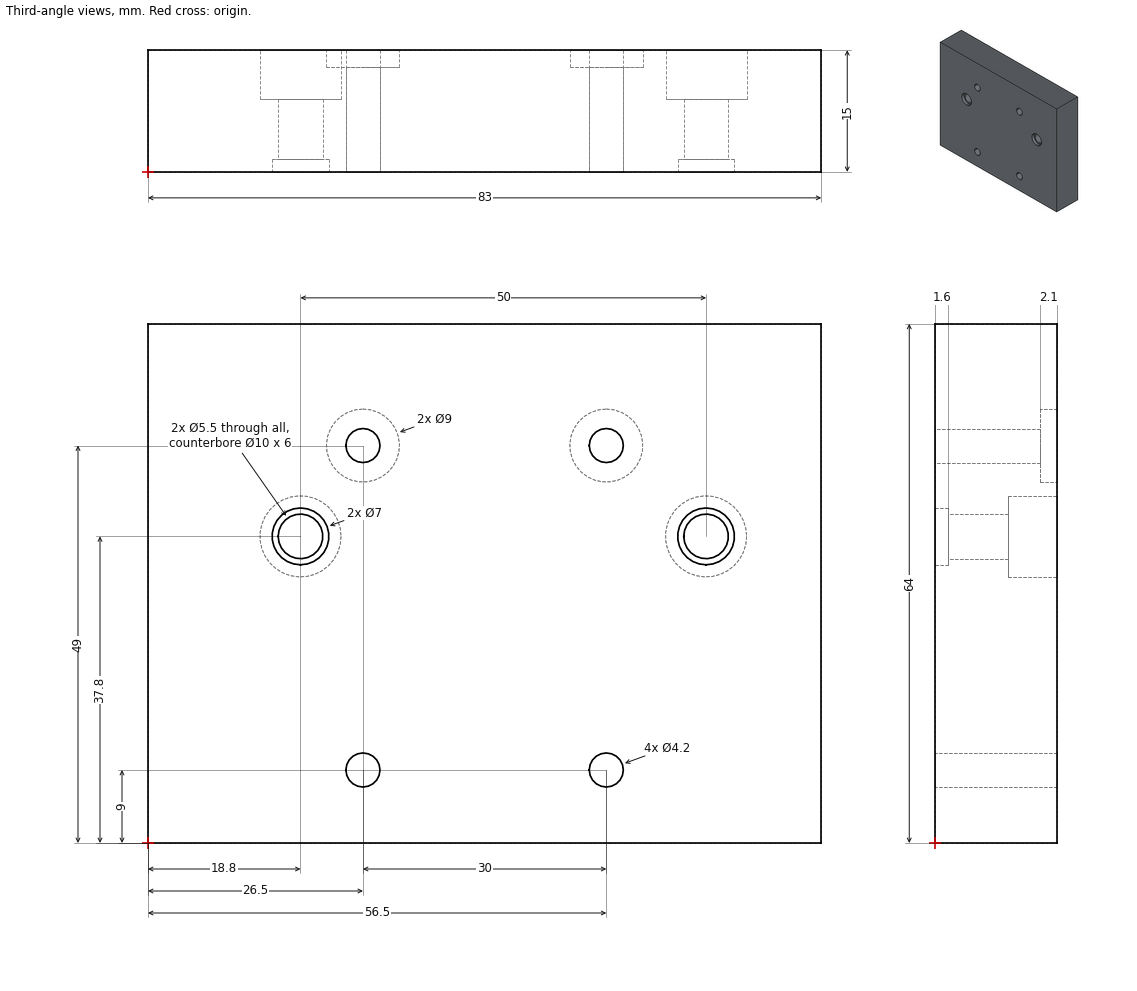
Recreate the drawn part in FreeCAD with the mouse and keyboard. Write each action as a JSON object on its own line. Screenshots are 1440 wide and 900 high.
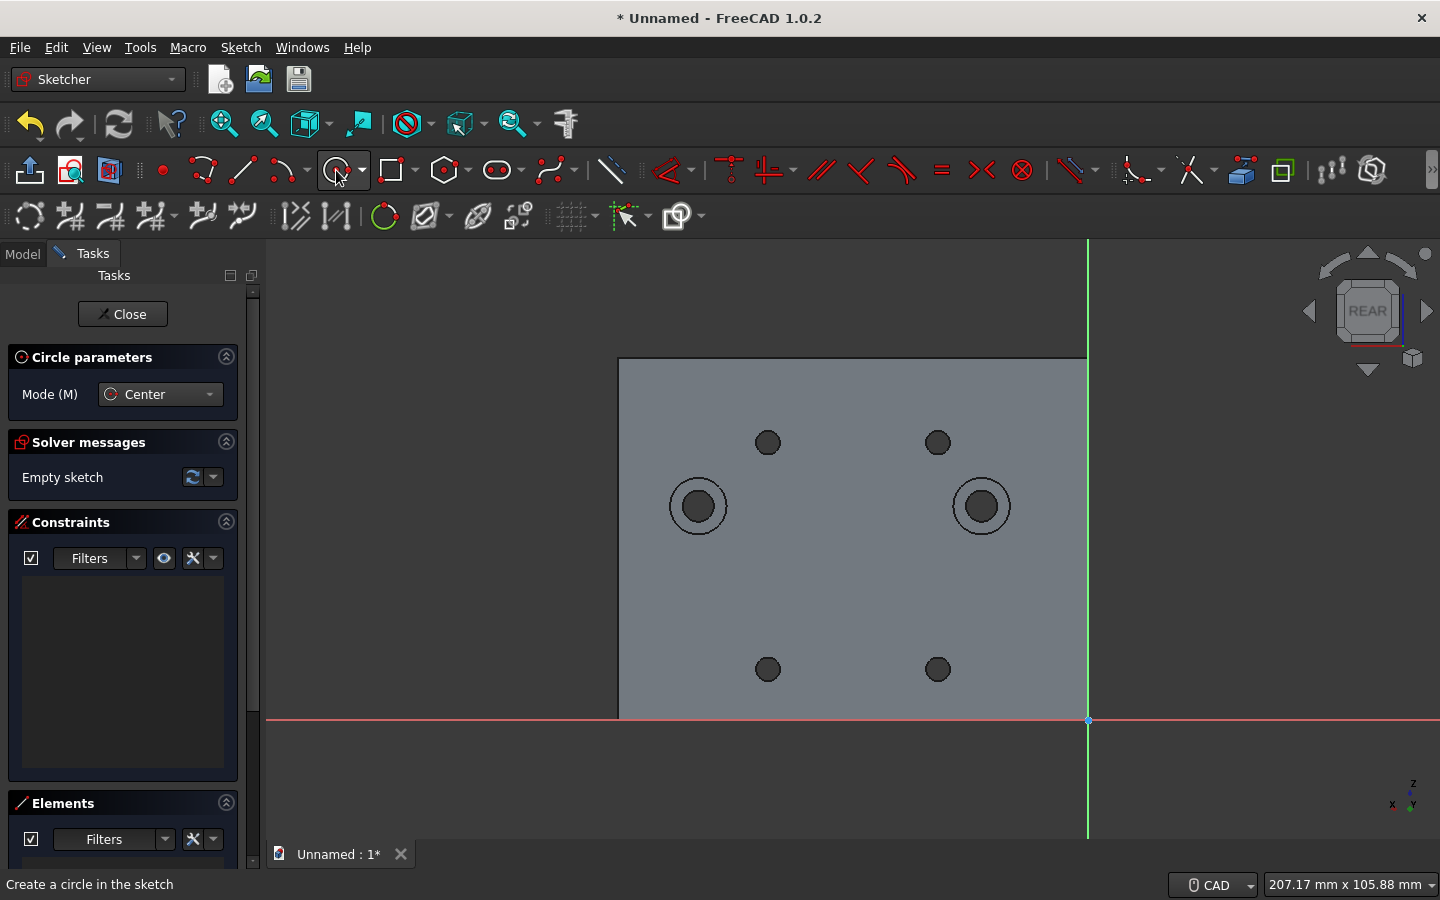
{"action": "left_click", "coordinate": [938, 443]}
{"action": "left_click", "coordinate": [956, 425]}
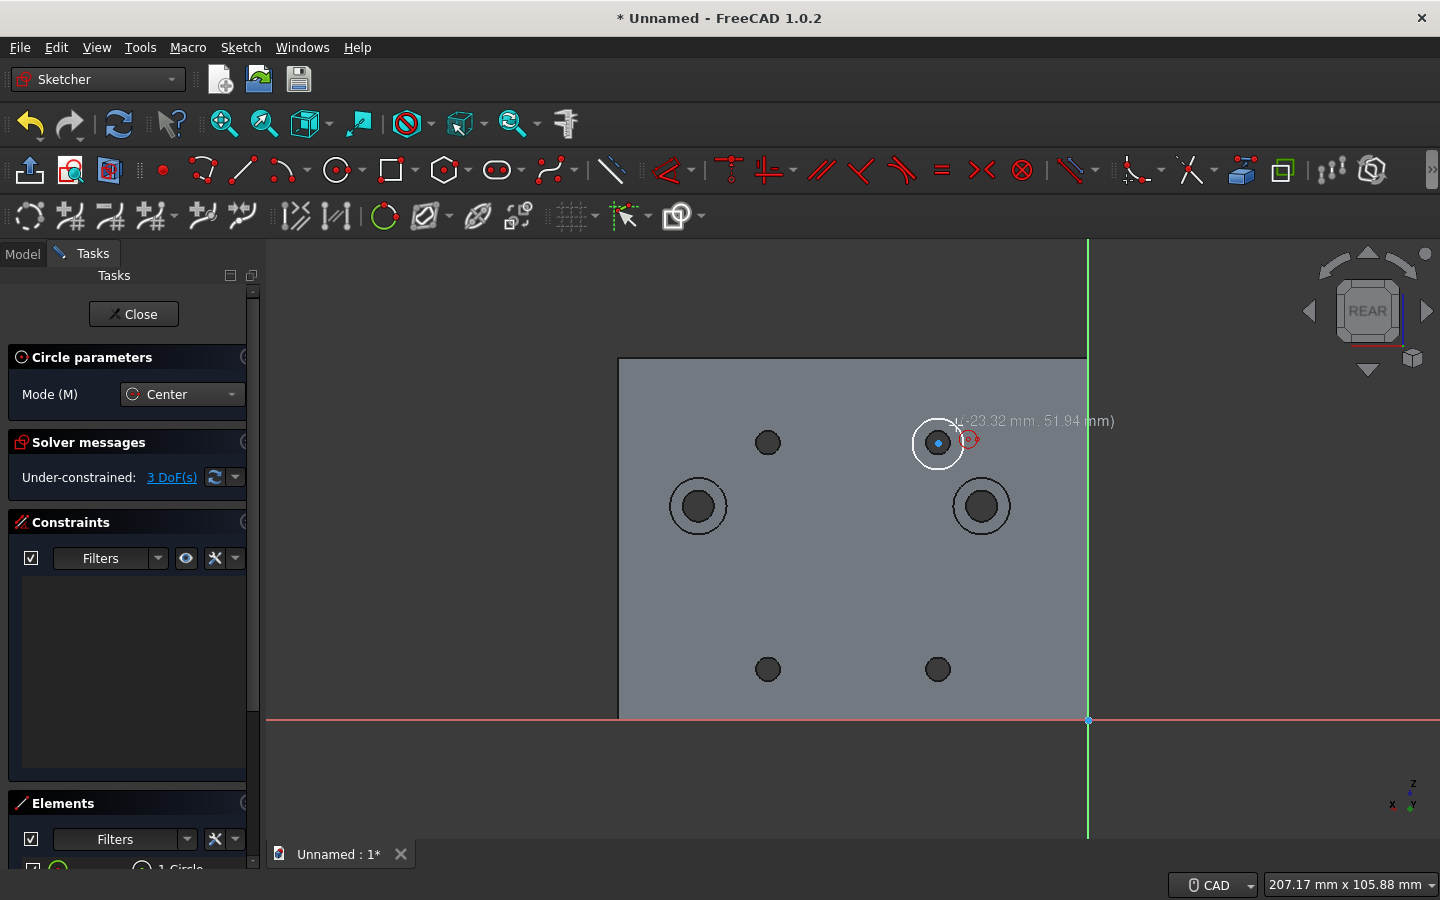
{"action": "left_click", "coordinate": [768, 443]}
{"action": "left_click", "coordinate": [786, 425]}
{"action": "key", "text": "Escape"}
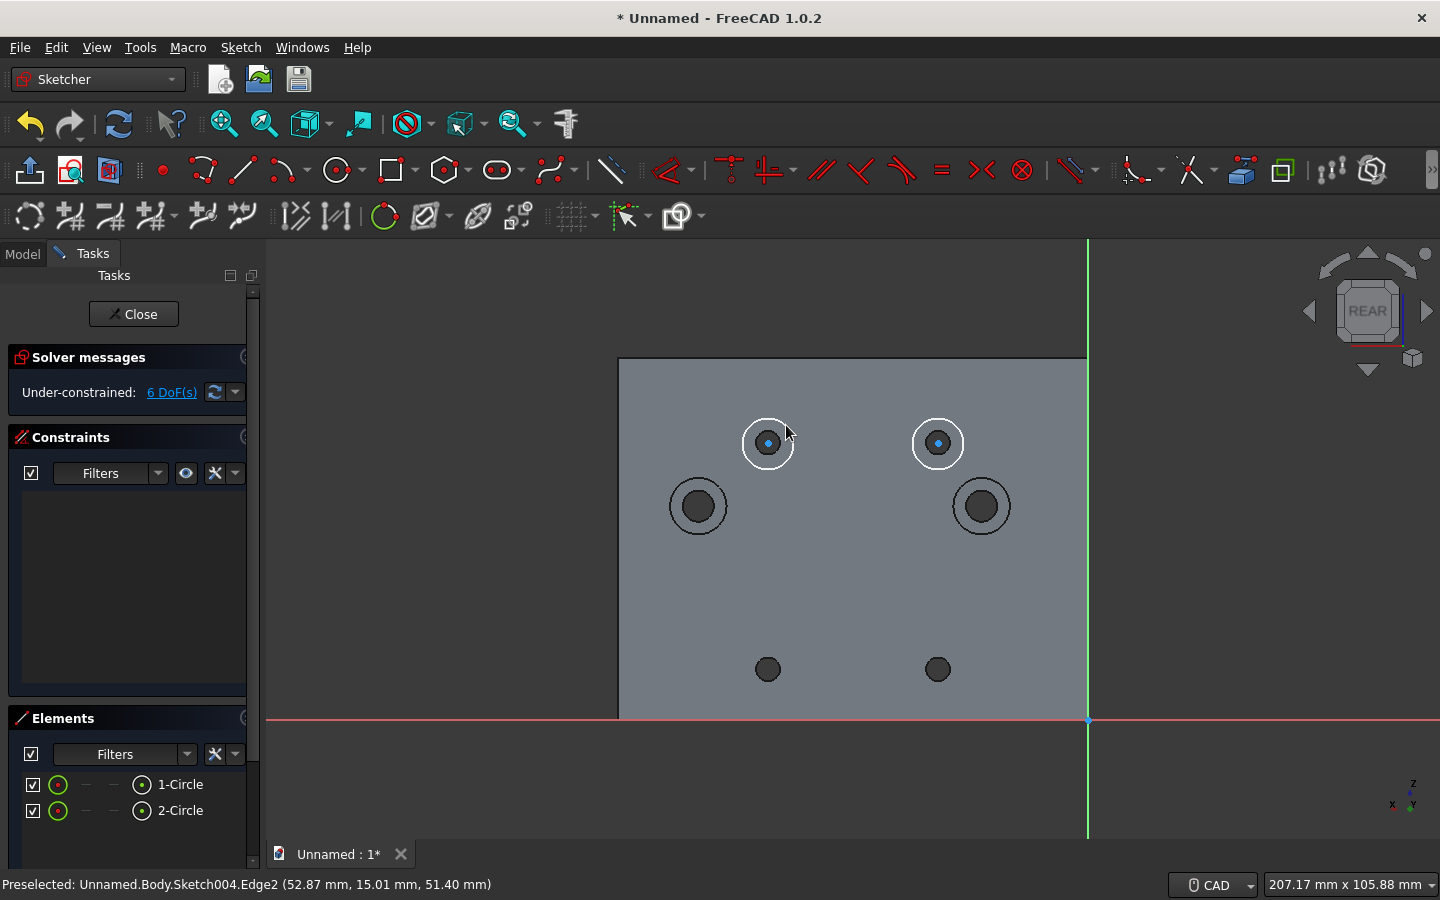
{"action": "left_click", "coordinate": [956, 426]}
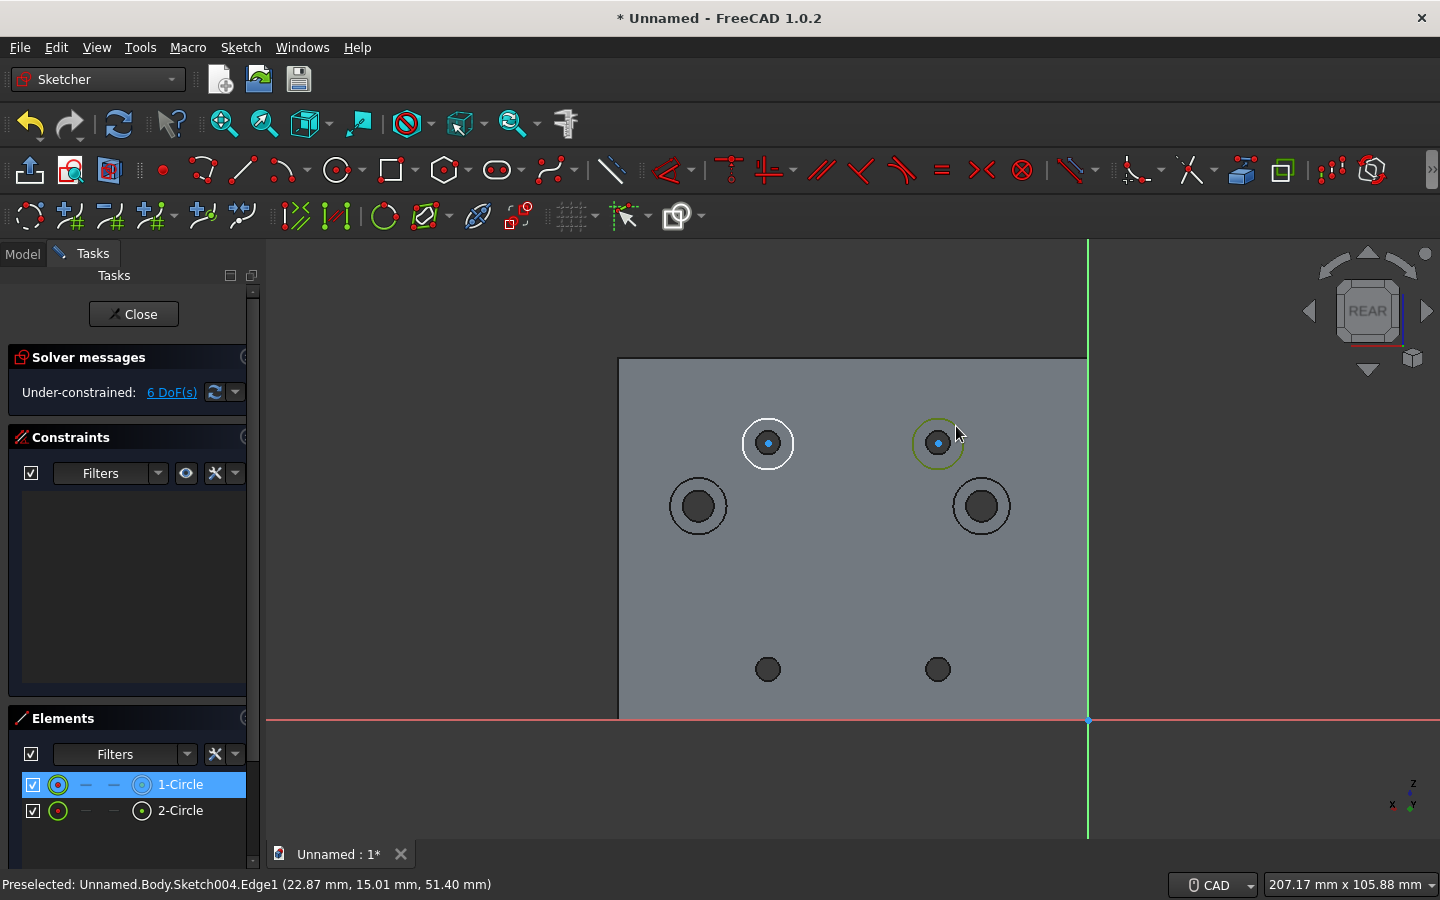
{"action": "left_click", "coordinate": [786, 426]}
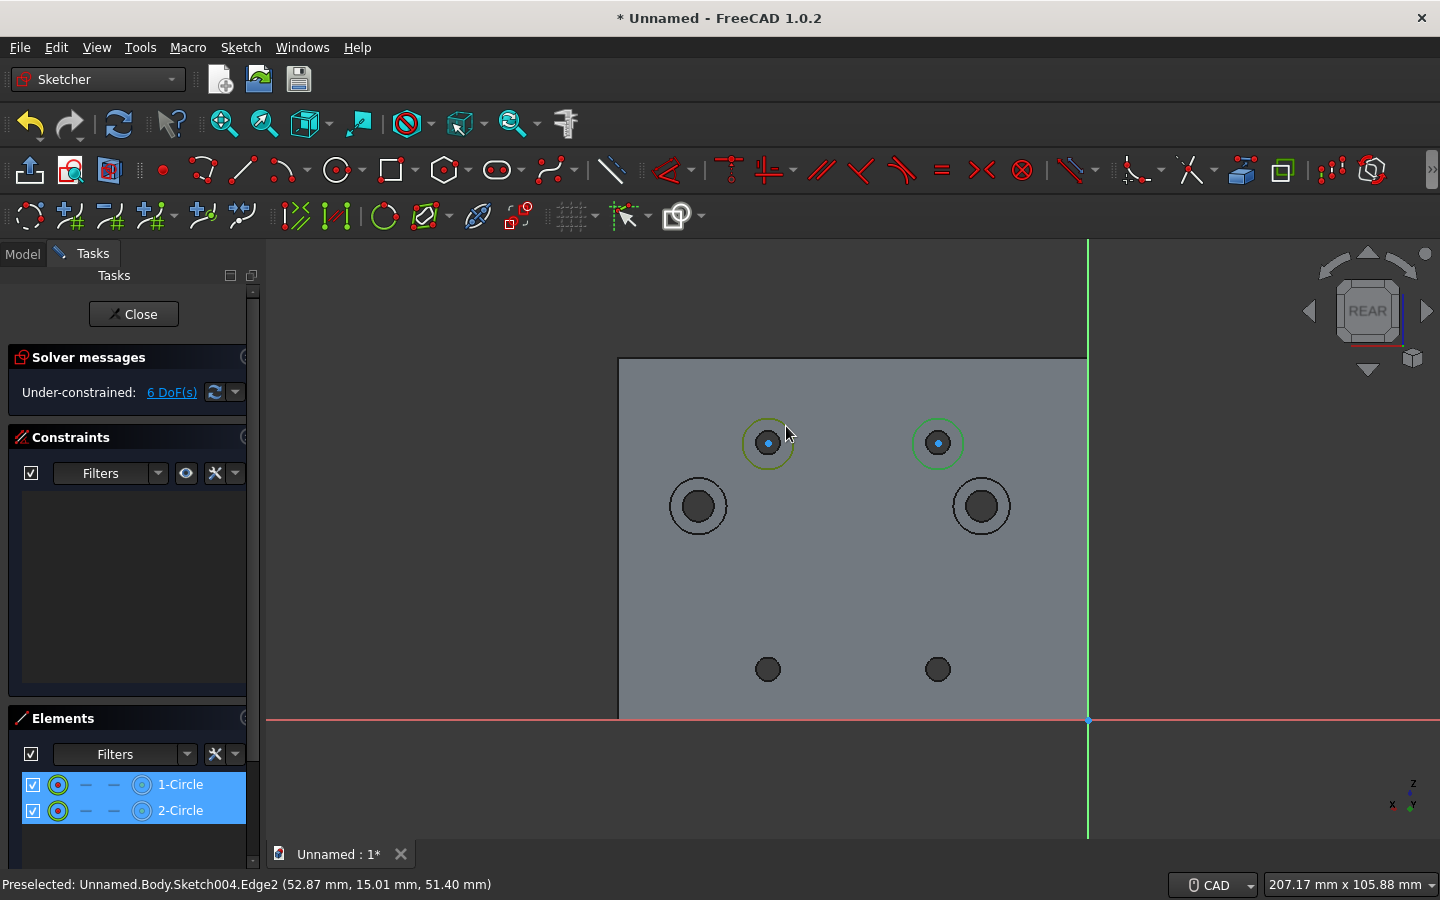
{"action": "left_click", "coordinate": [942, 170]}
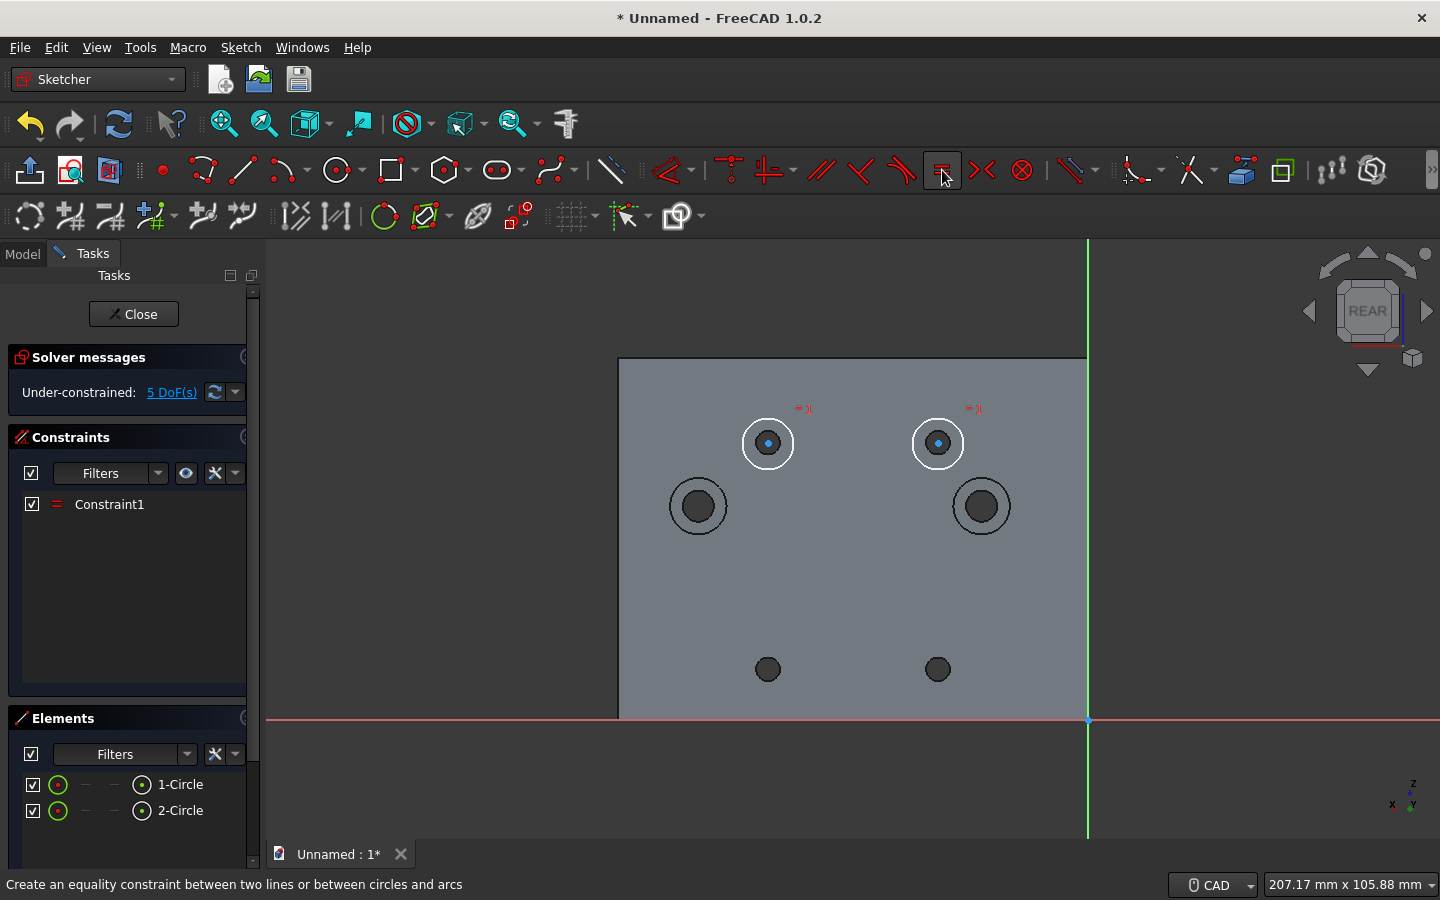
{"action": "left_click", "coordinate": [666, 170]}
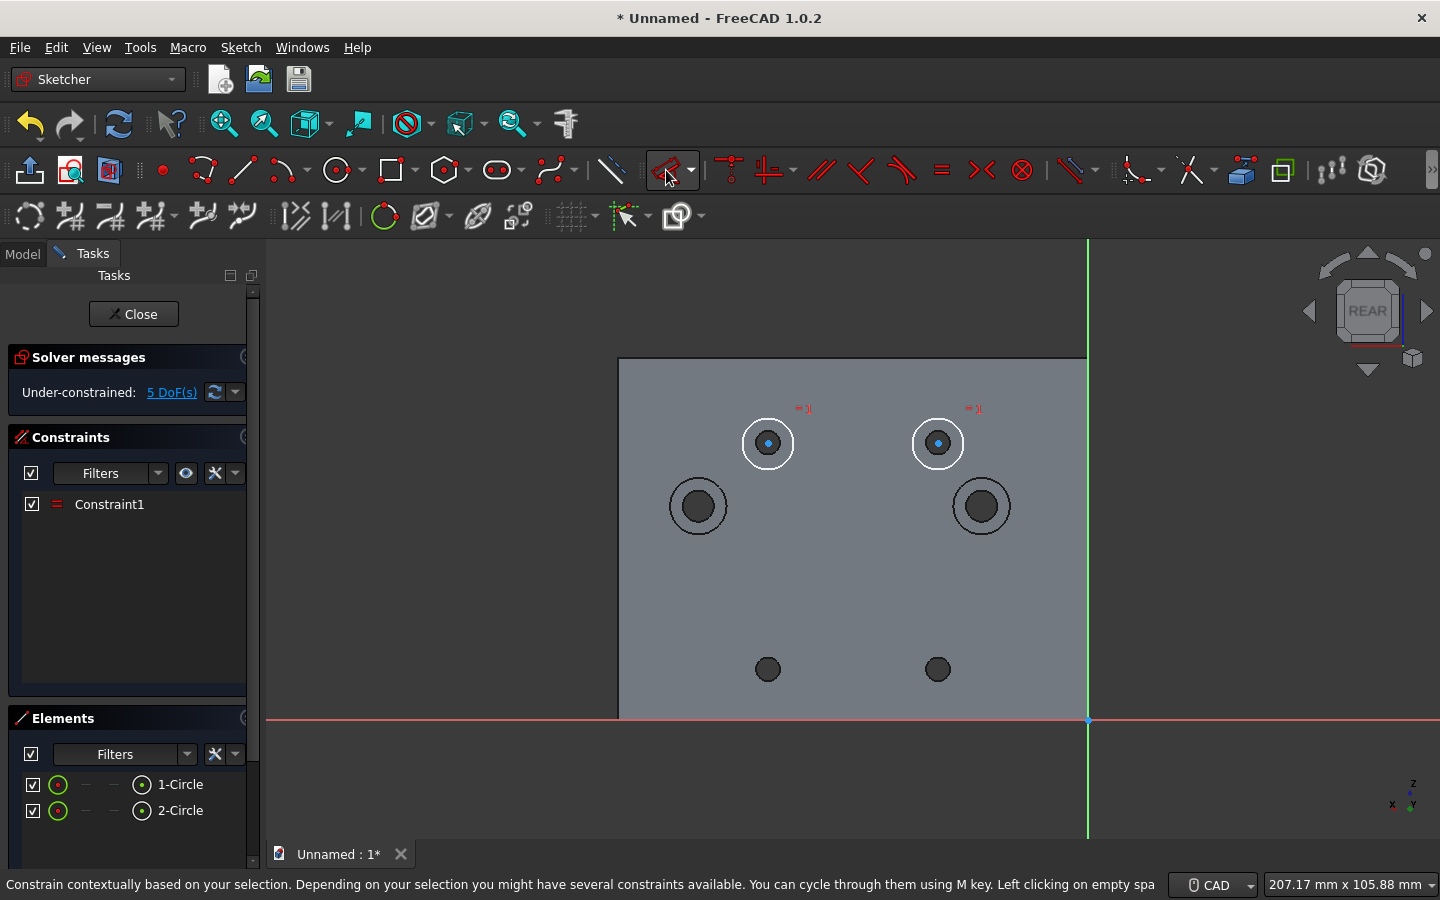
{"action": "left_click", "coordinate": [956, 426]}
{"action": "left_click", "coordinate": [979, 403]}